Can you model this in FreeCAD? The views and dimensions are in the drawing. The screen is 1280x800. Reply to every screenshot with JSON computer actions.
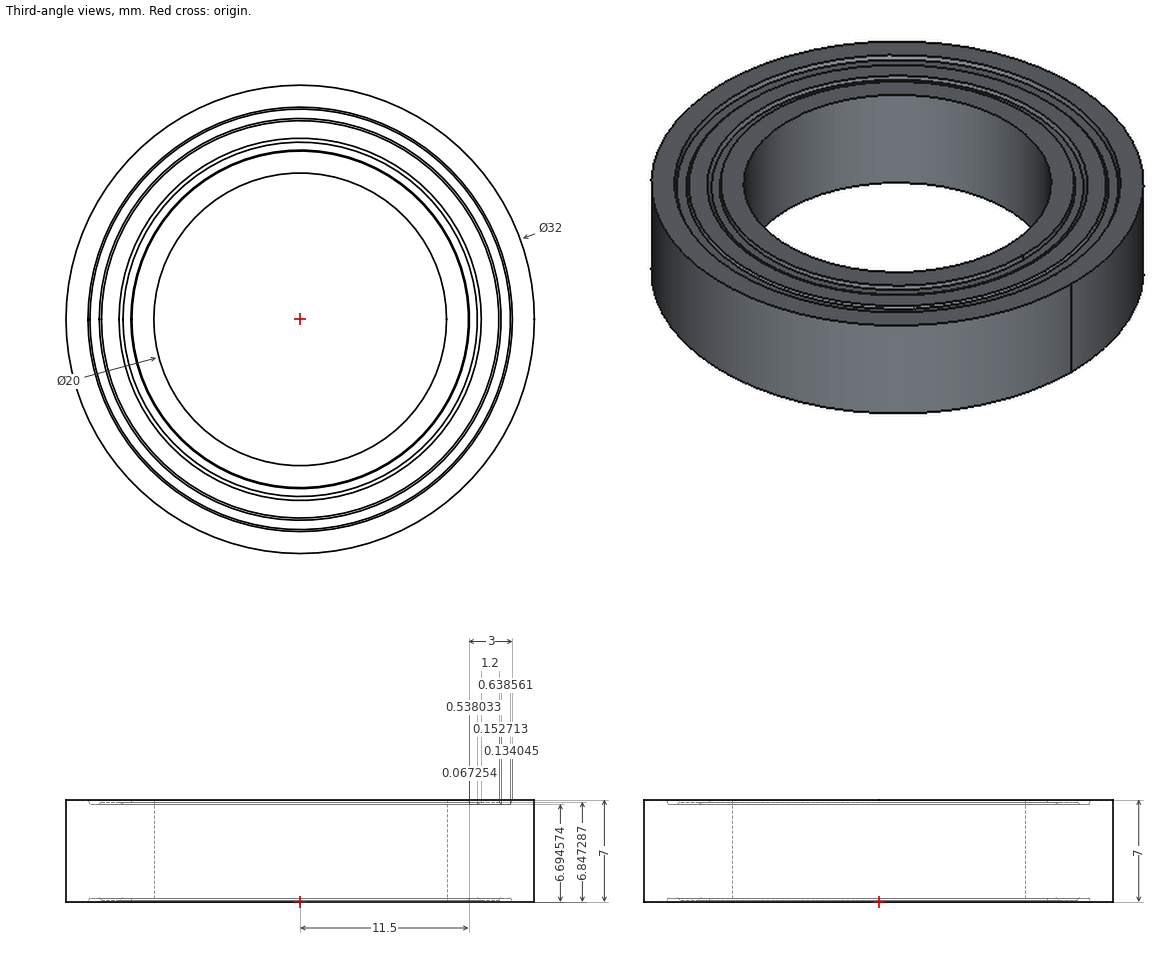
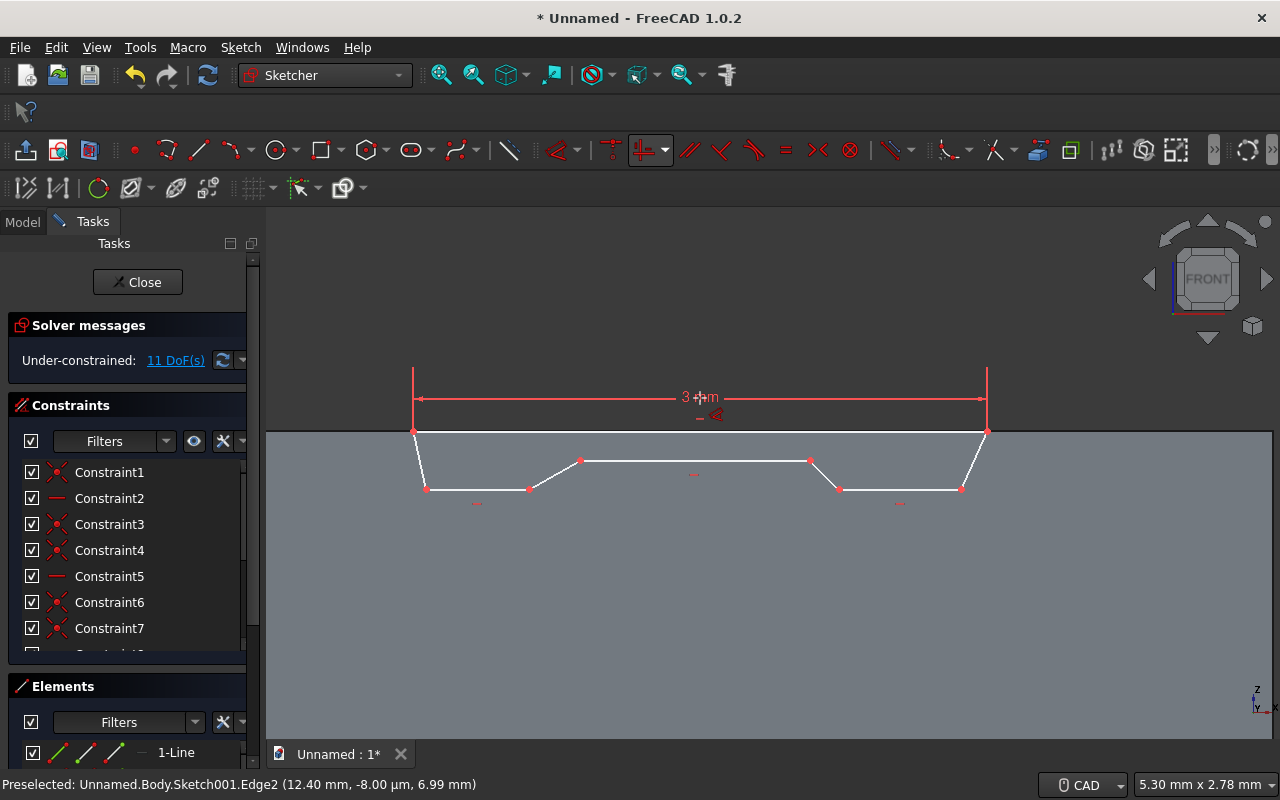
{"action": "left_click", "coordinate": [413, 432]}
{"action": "left_click", "coordinate": [447, 571]}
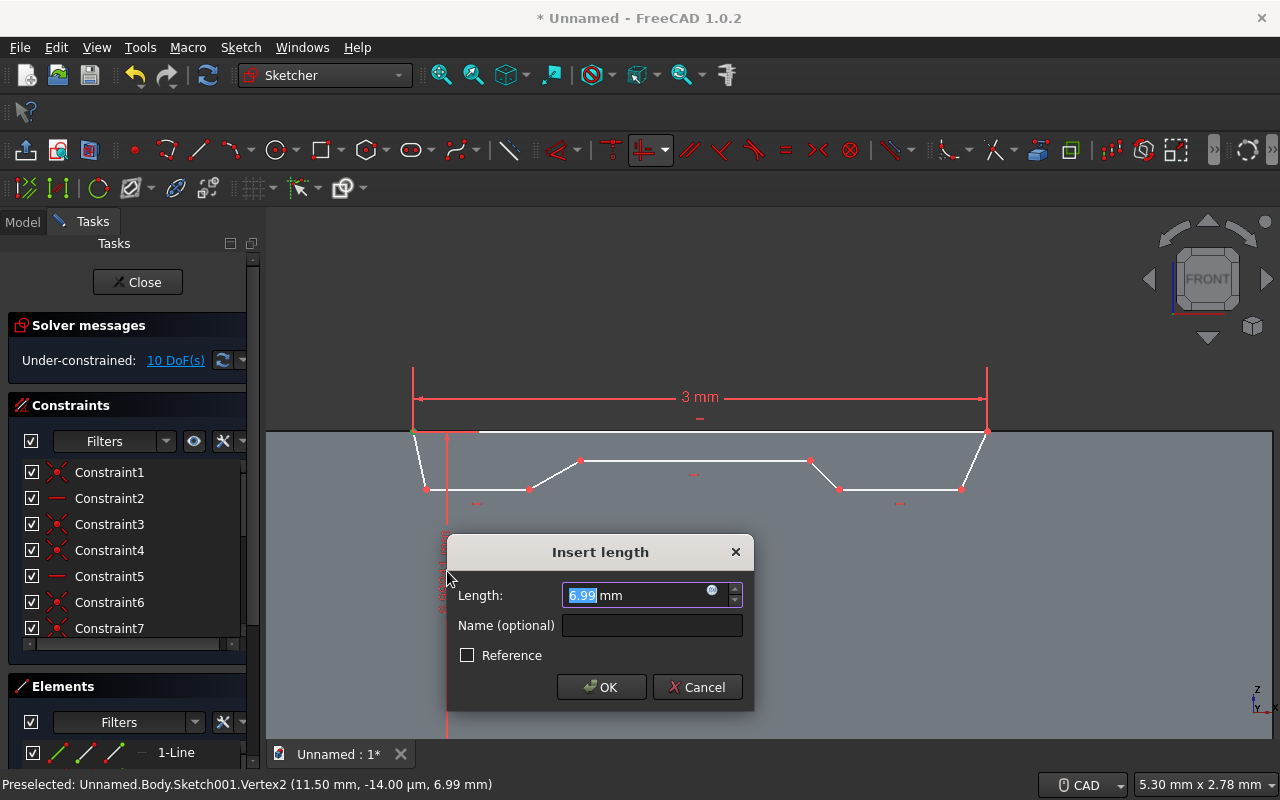
{"action": "type", "text": "7"}
{"action": "key", "text": "Return"}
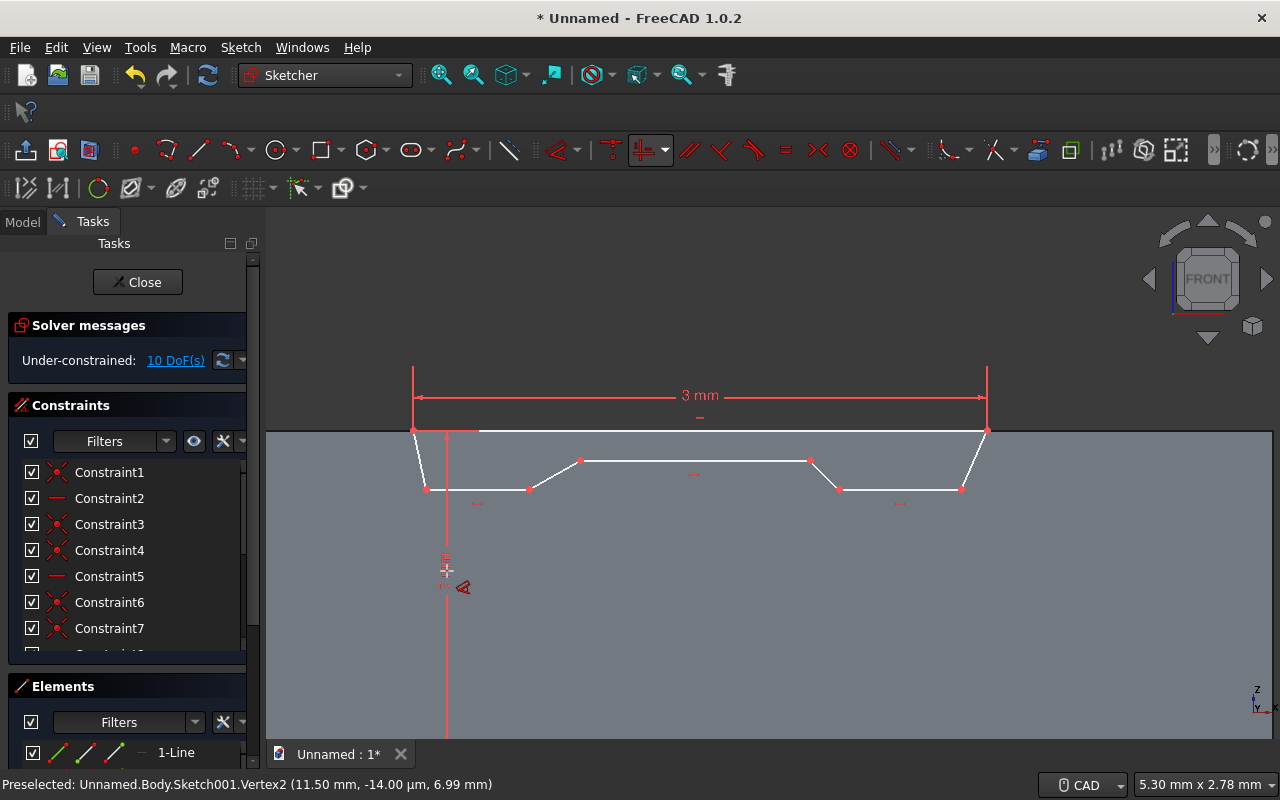
{"action": "left_click", "coordinate": [741, 461]}
{"action": "left_click", "coordinate": [695, 495]}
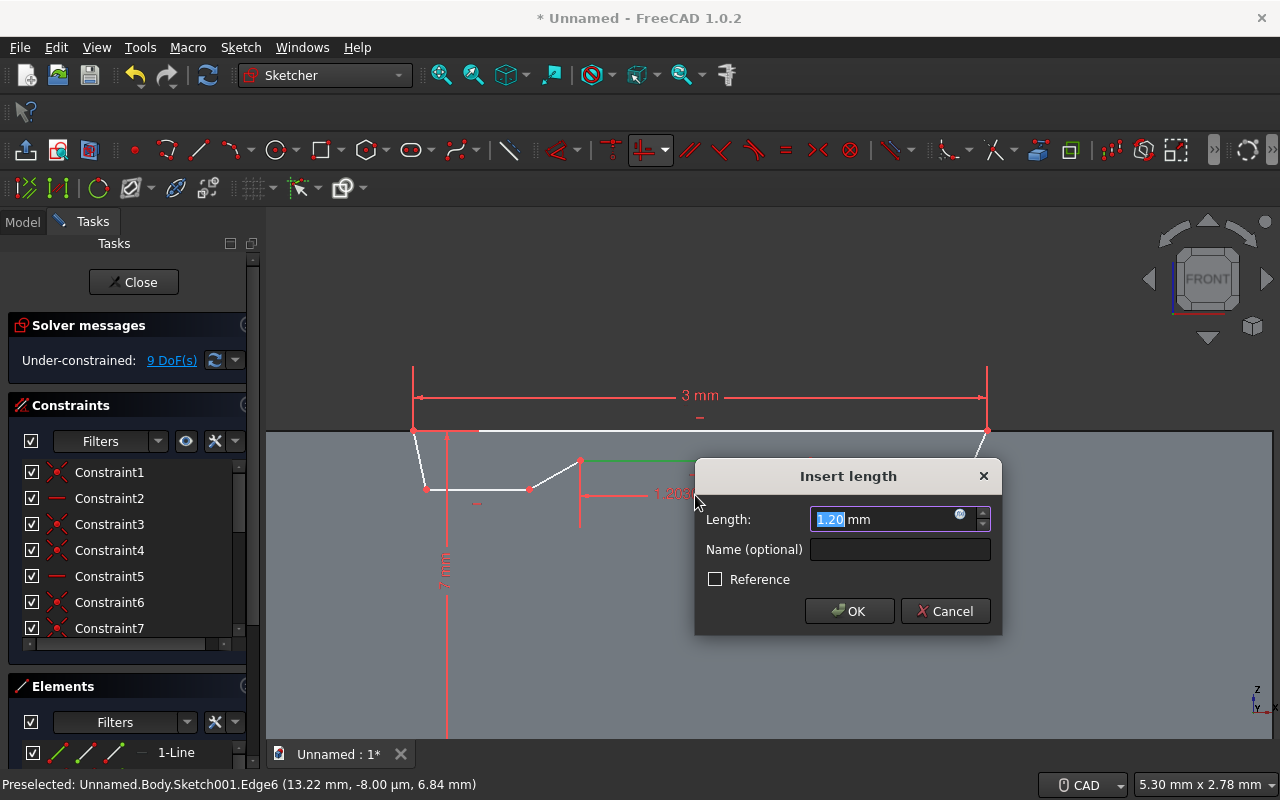
{"action": "type", "text": "1.2"}
{"action": "key", "text": "Return"}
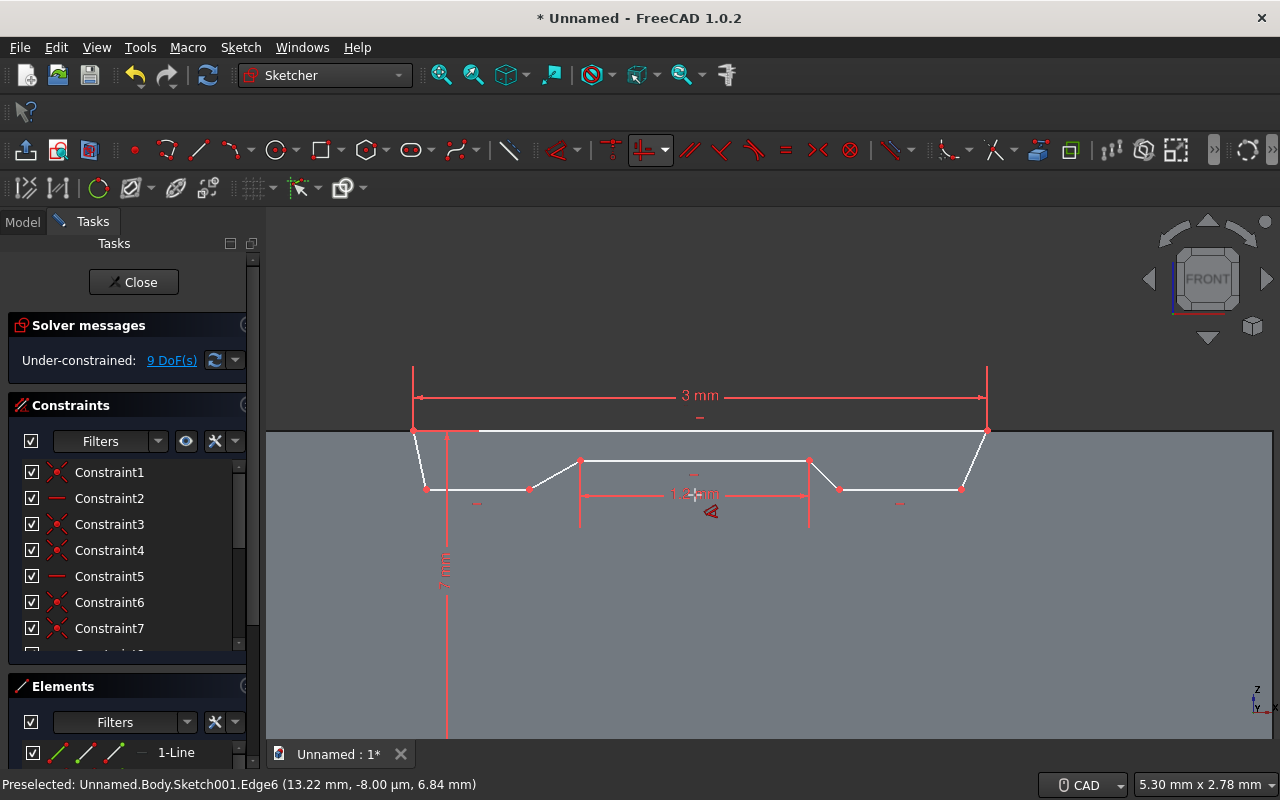
{"action": "left_click", "coordinate": [413, 431]}
{"action": "left_click", "coordinate": [354, 397]}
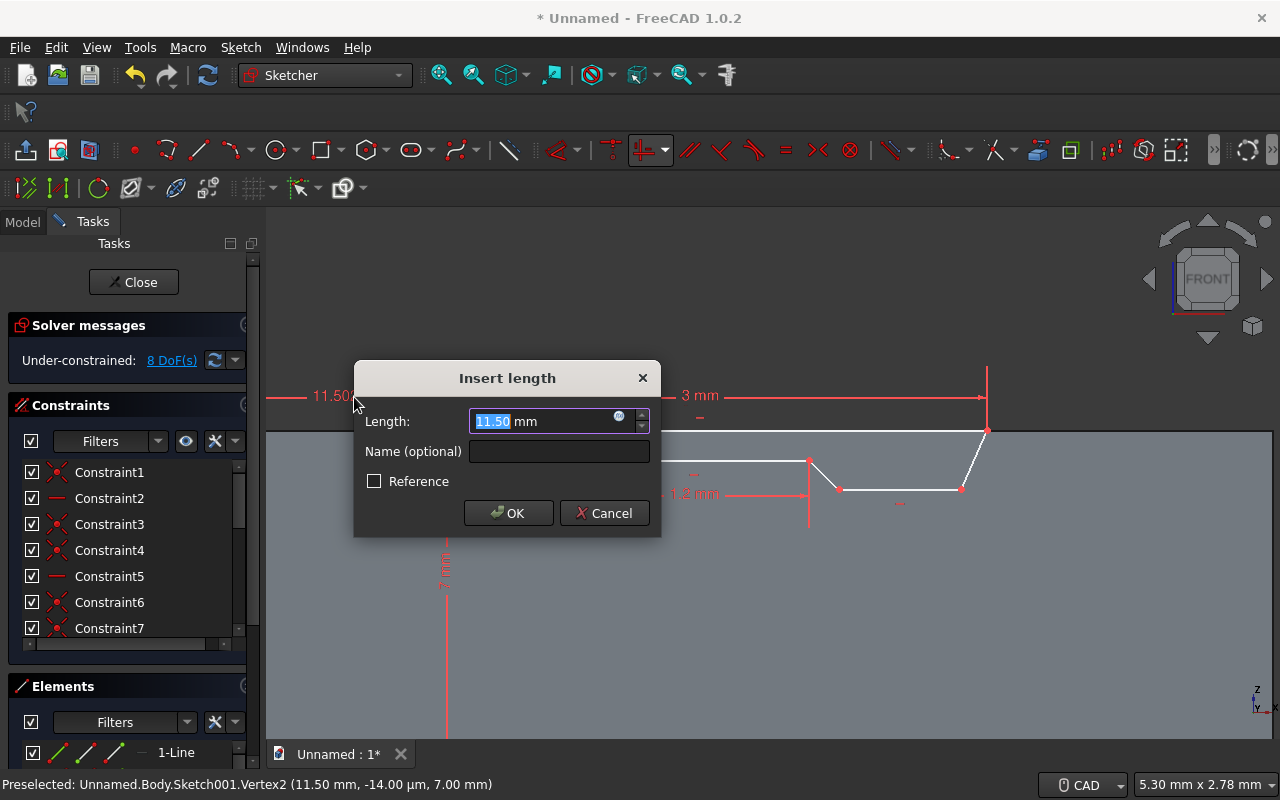
{"action": "type", "text": "11.5"}
{"action": "key", "text": "Return"}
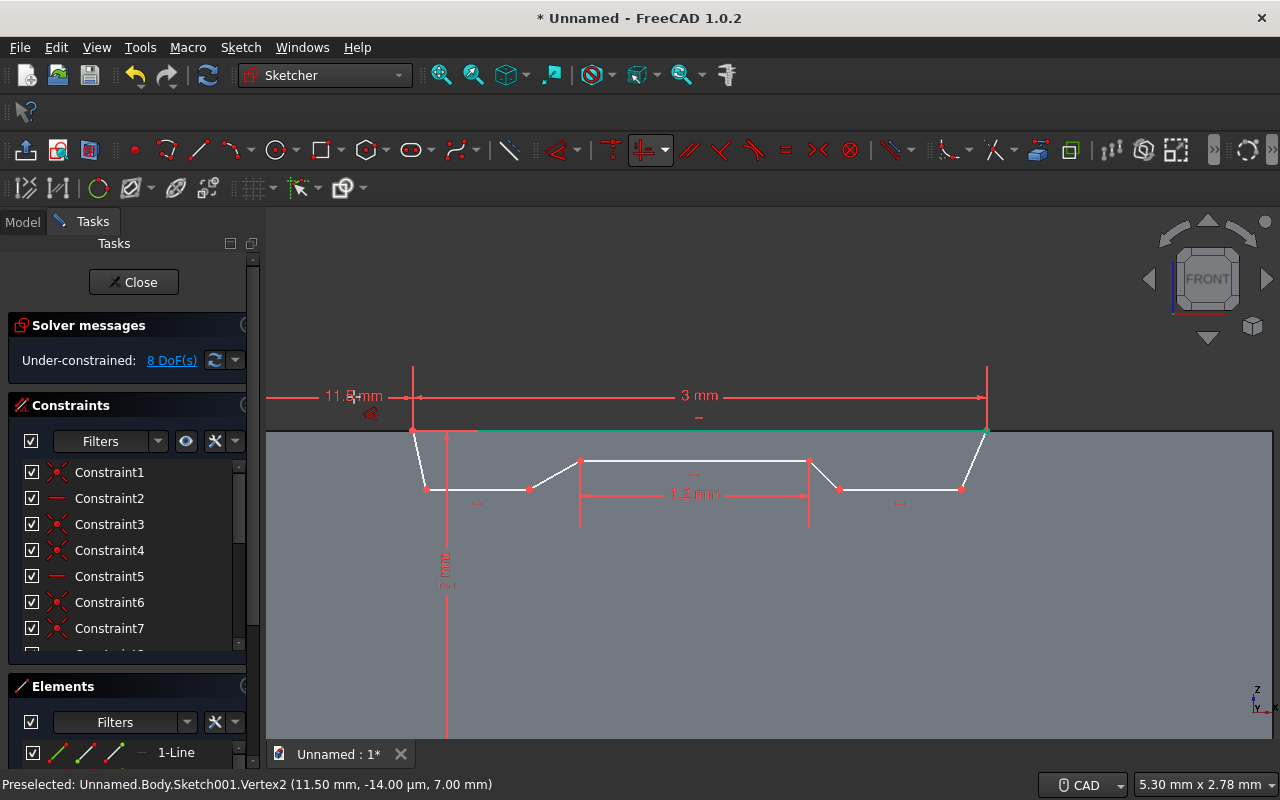
{"action": "left_click", "coordinate": [924, 490]}
{"action": "left_click", "coordinate": [900, 524]}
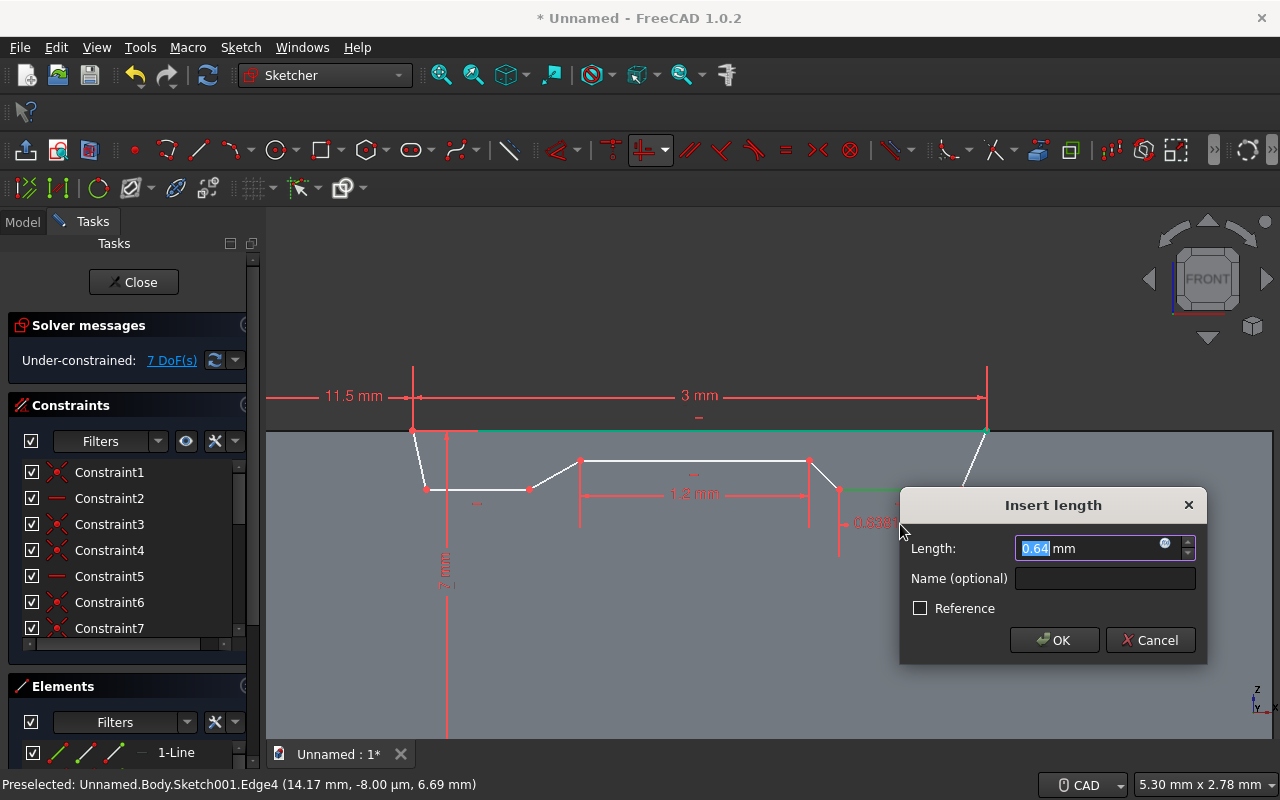
{"action": "type", "text": "0.638561"}
{"action": "key", "text": "Return"}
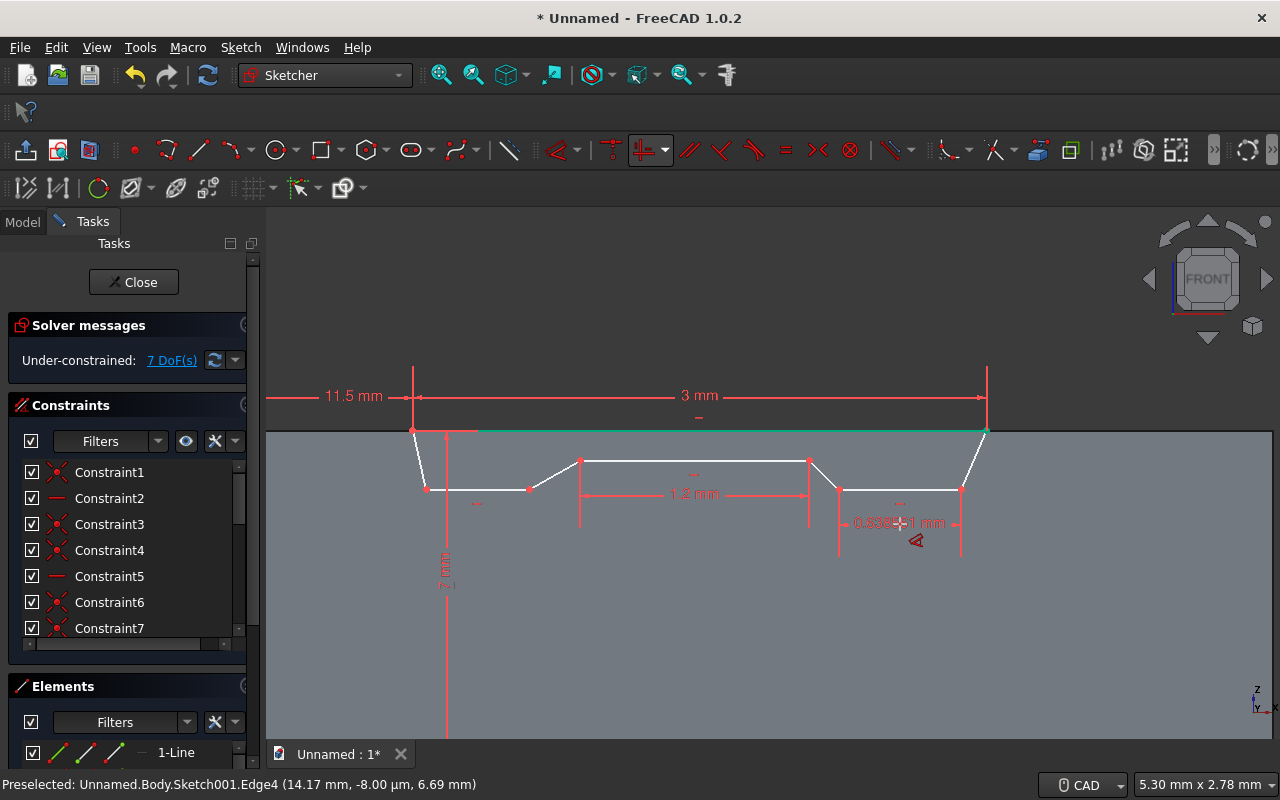
{"action": "left_click", "coordinate": [498, 490]}
{"action": "left_click", "coordinate": [478, 524]}